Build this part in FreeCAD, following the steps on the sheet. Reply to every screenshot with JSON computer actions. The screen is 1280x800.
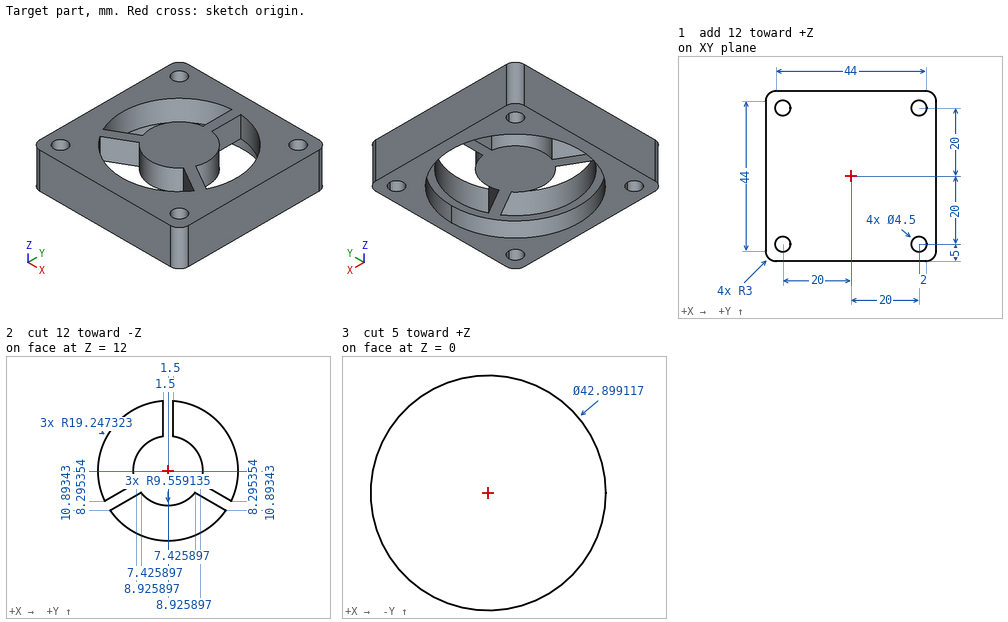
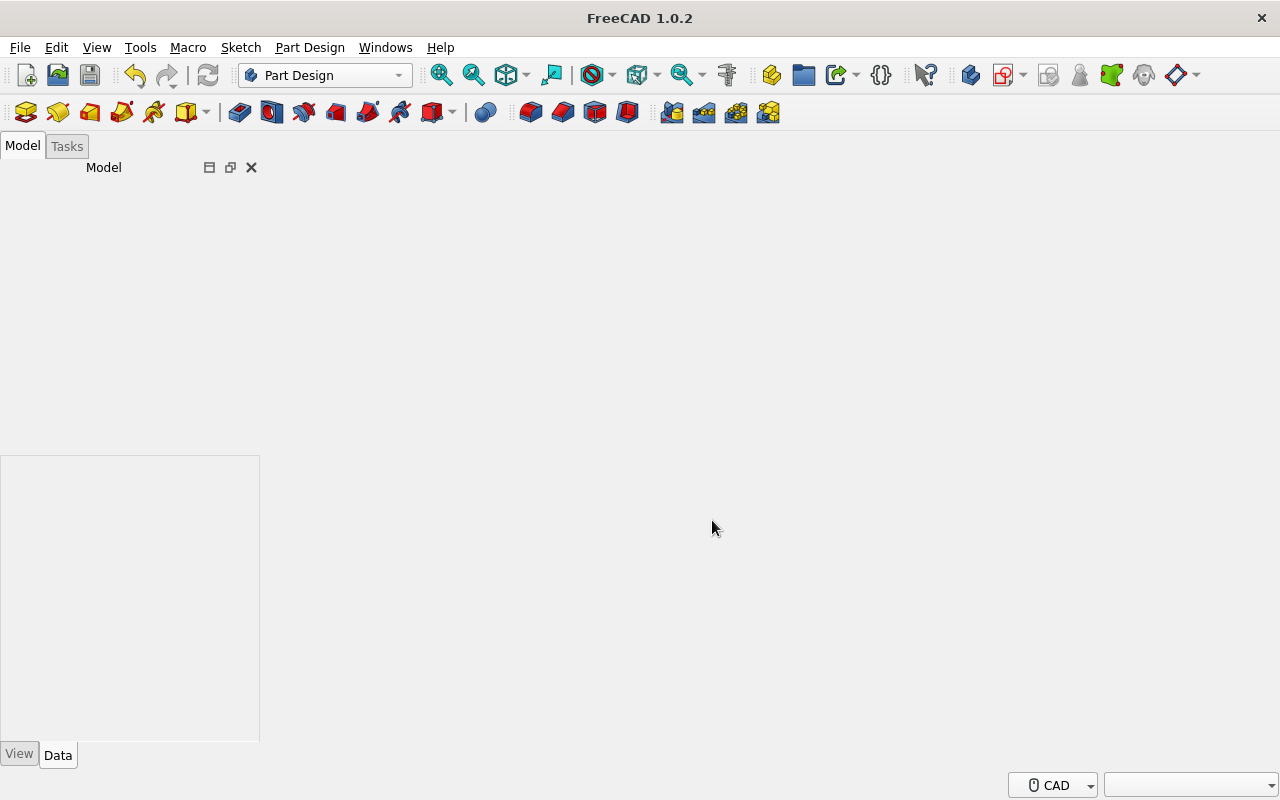
{"action": "left_click", "coordinate": [26, 76]}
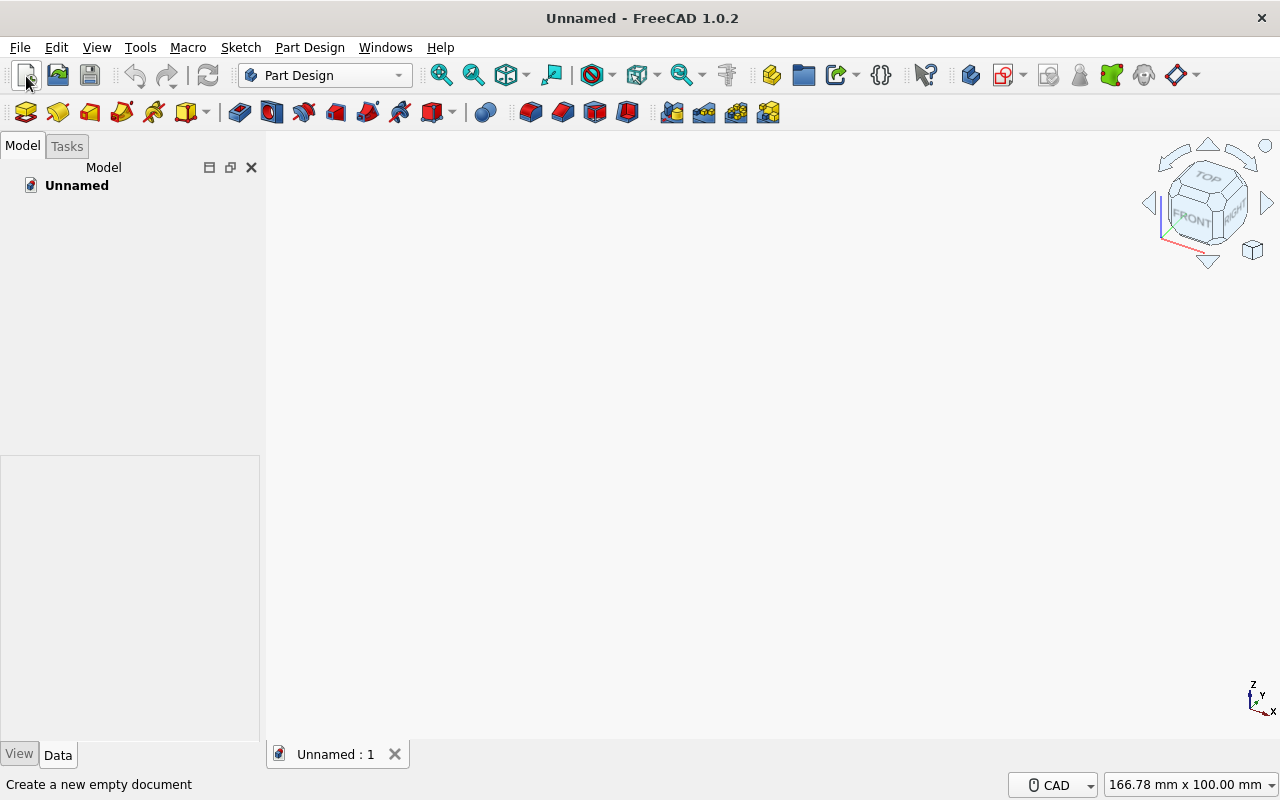
{"action": "left_click", "coordinate": [1004, 76]}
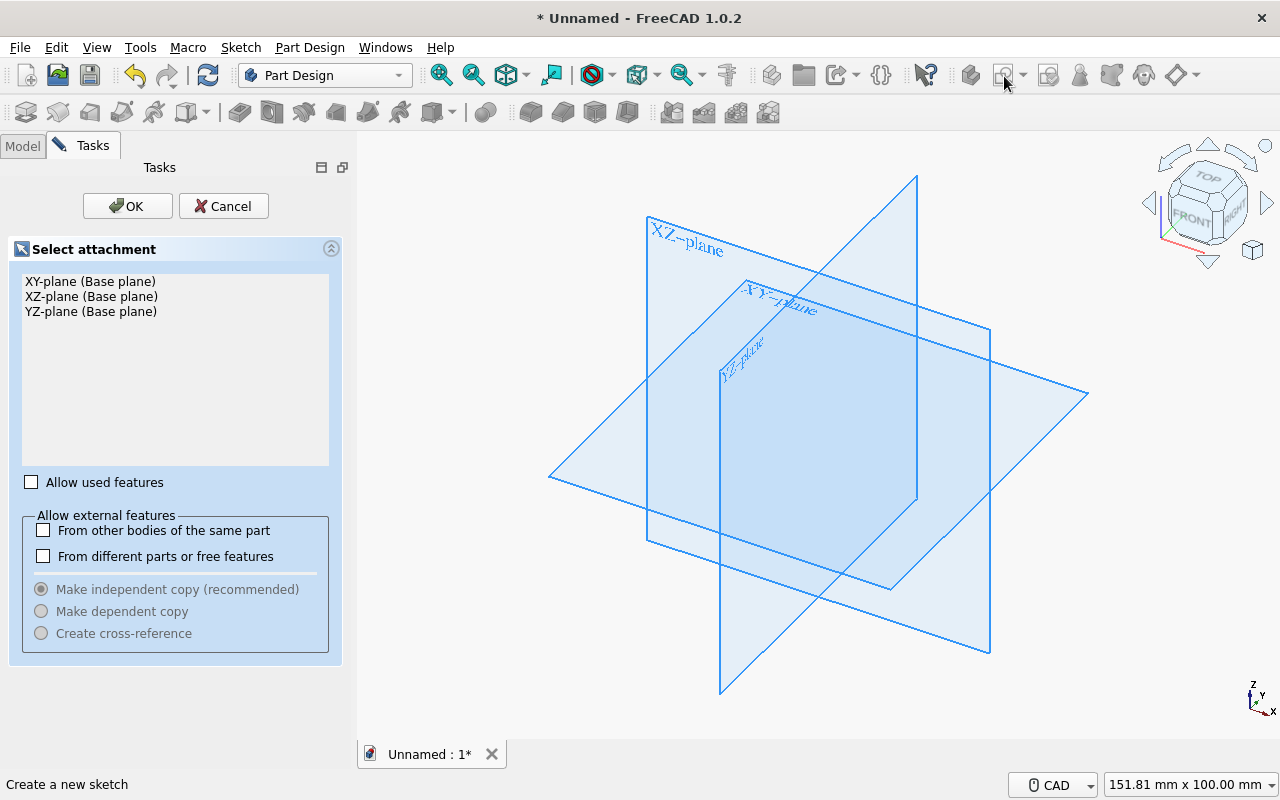
{"action": "left_click", "coordinate": [82, 282]}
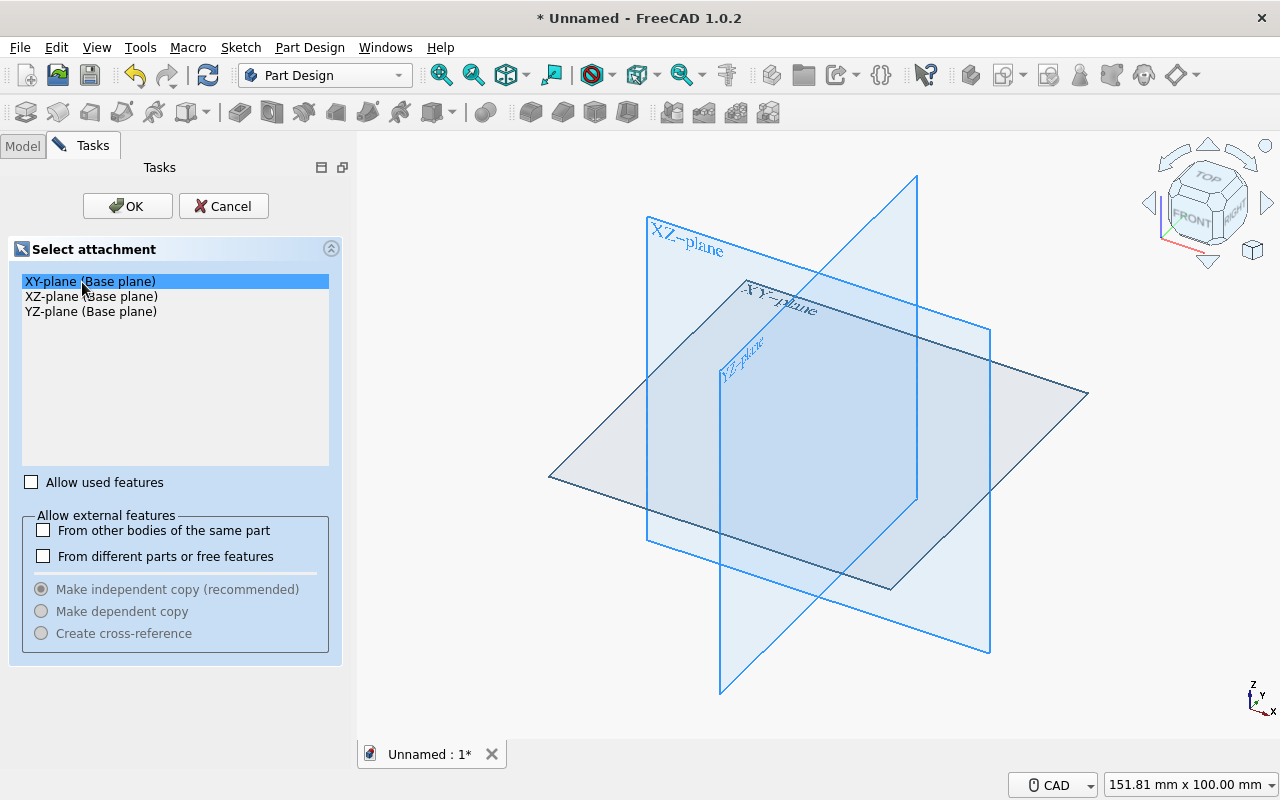
{"action": "left_click", "coordinate": [128, 206]}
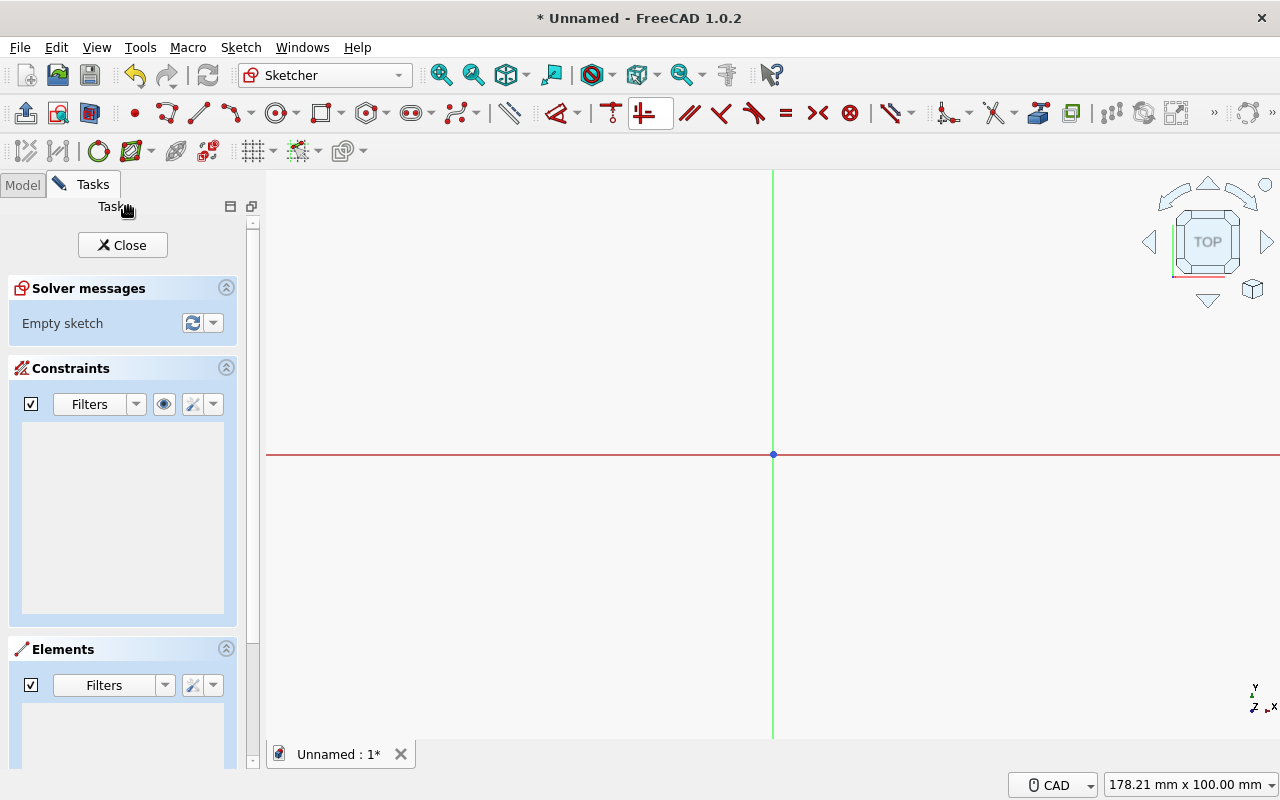
{"action": "left_click", "coordinate": [200, 114]}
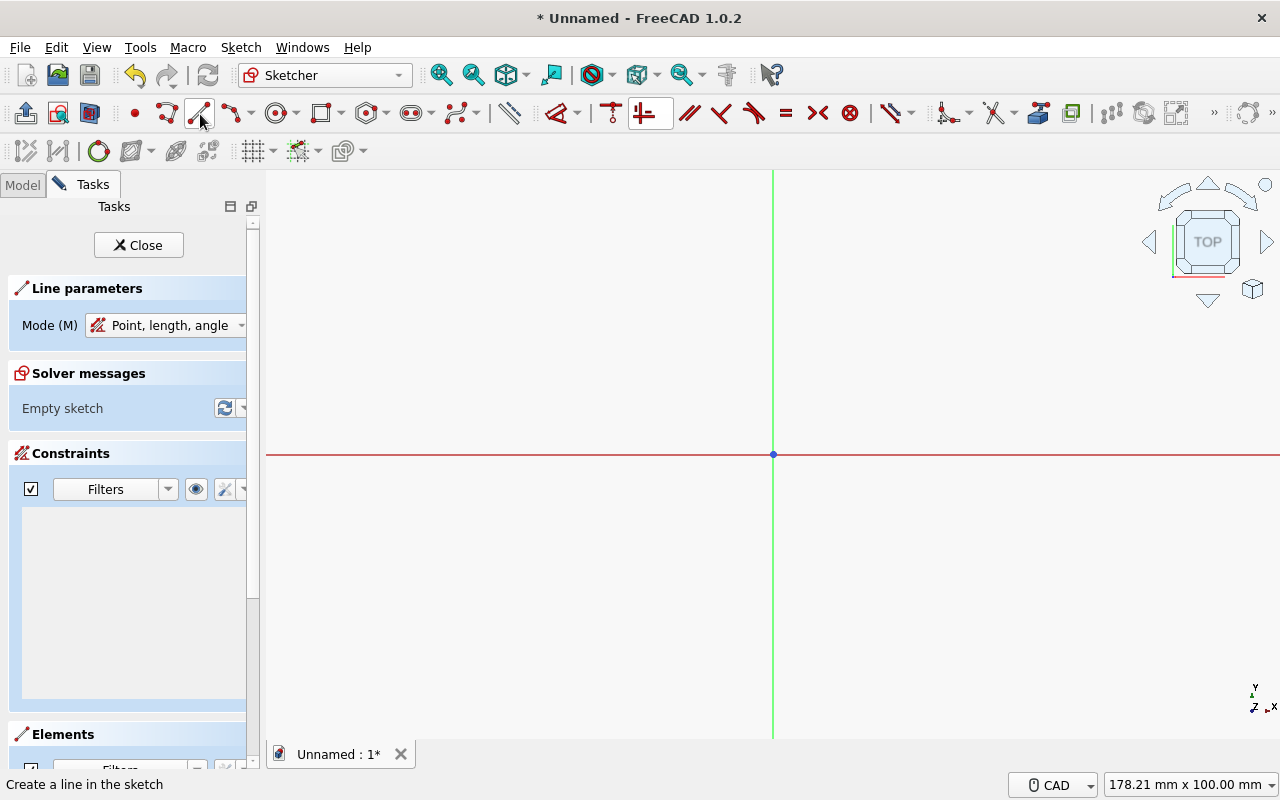
{"action": "left_click", "coordinate": [898, 312]}
{"action": "left_click", "coordinate": [648, 312]}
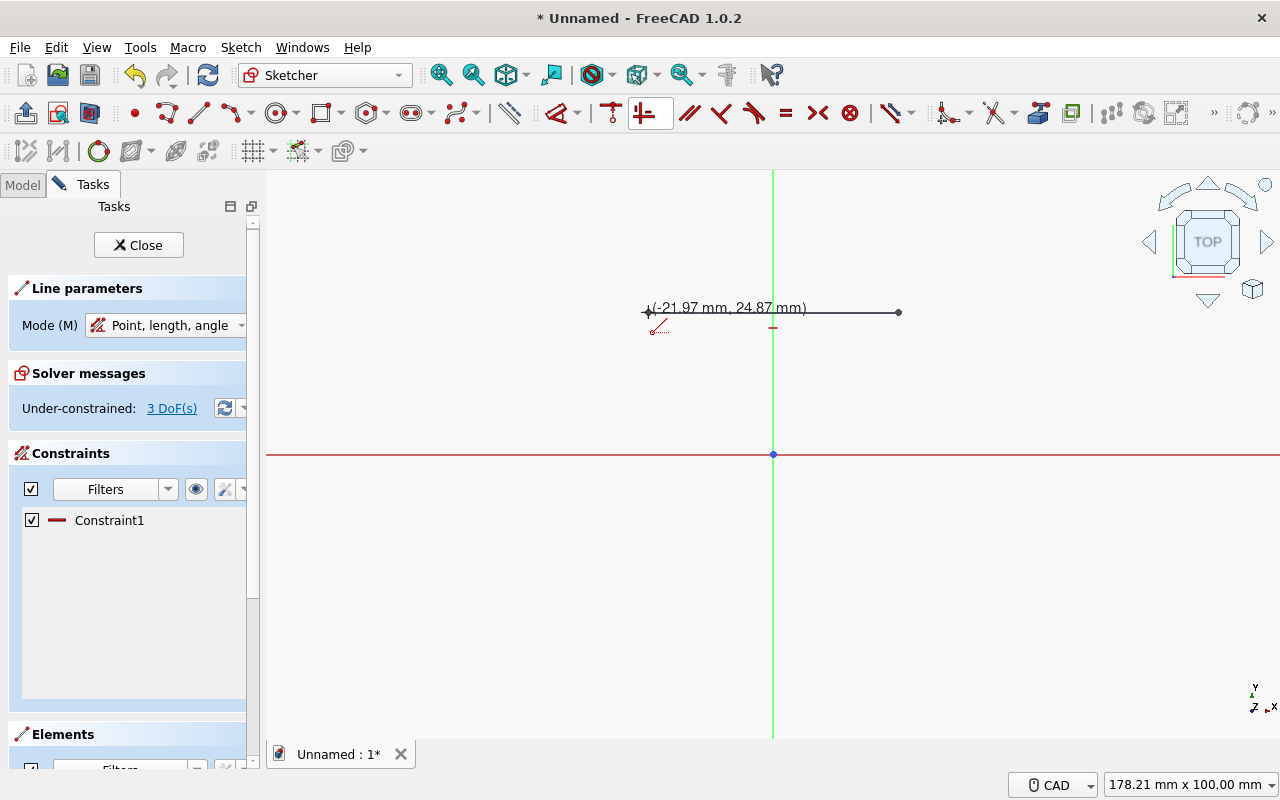
{"action": "left_click", "coordinate": [631, 329]}
{"action": "left_click", "coordinate": [631, 580]}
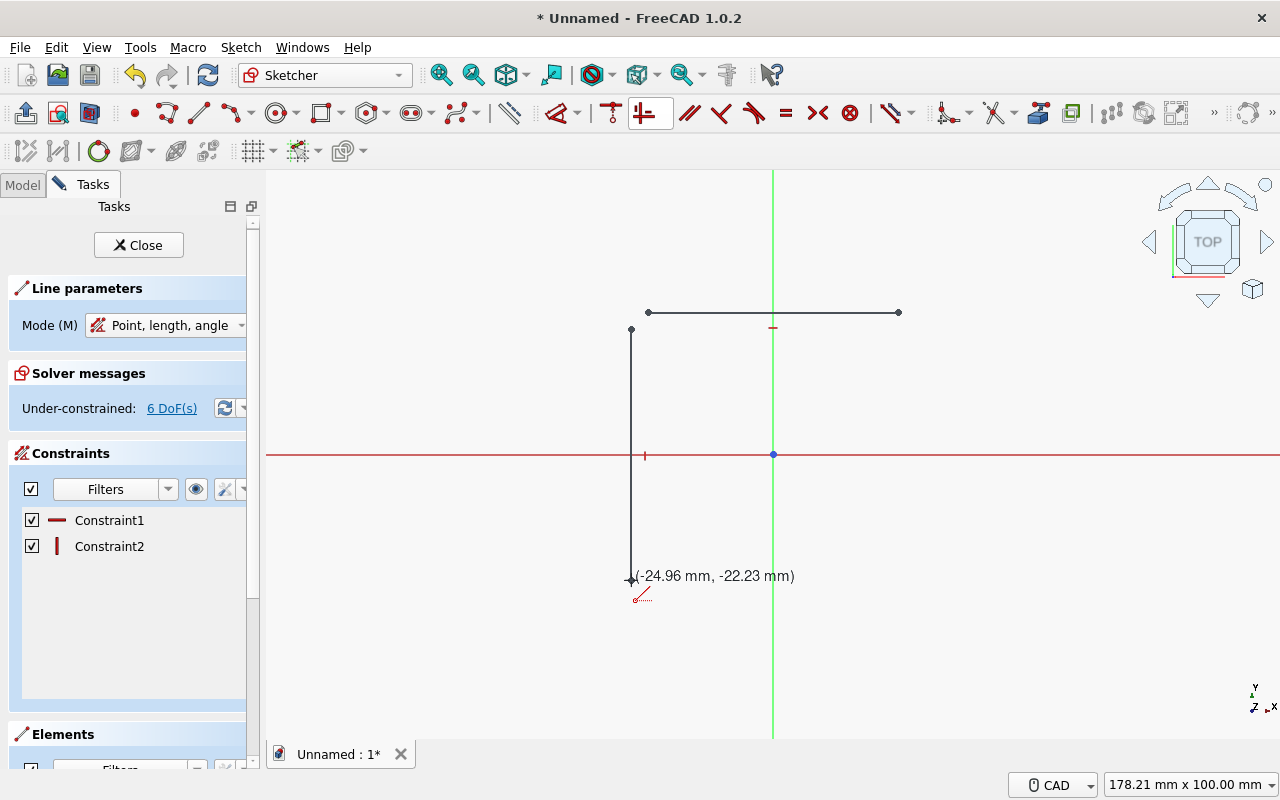
{"action": "left_click", "coordinate": [648, 597]}
{"action": "left_click", "coordinate": [898, 597]}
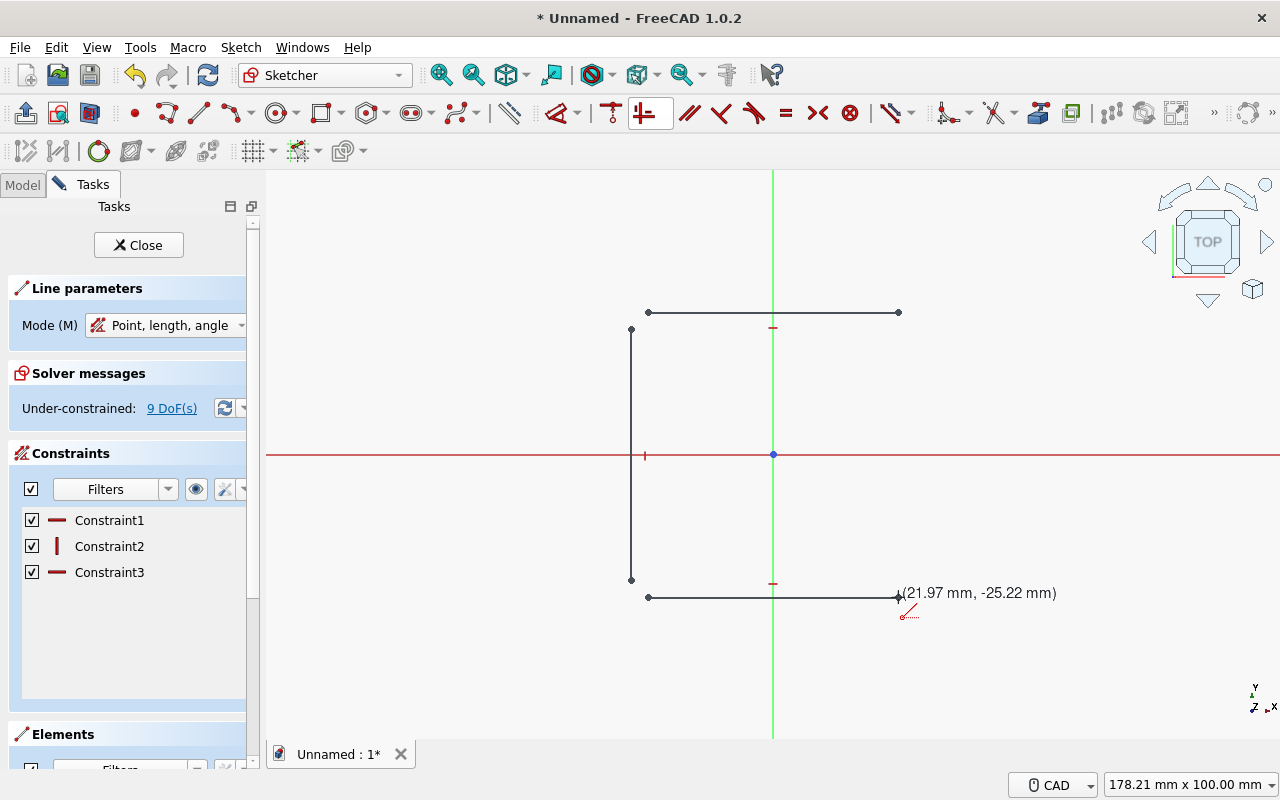
{"action": "left_click", "coordinate": [915, 580]}
{"action": "left_click", "coordinate": [915, 329]}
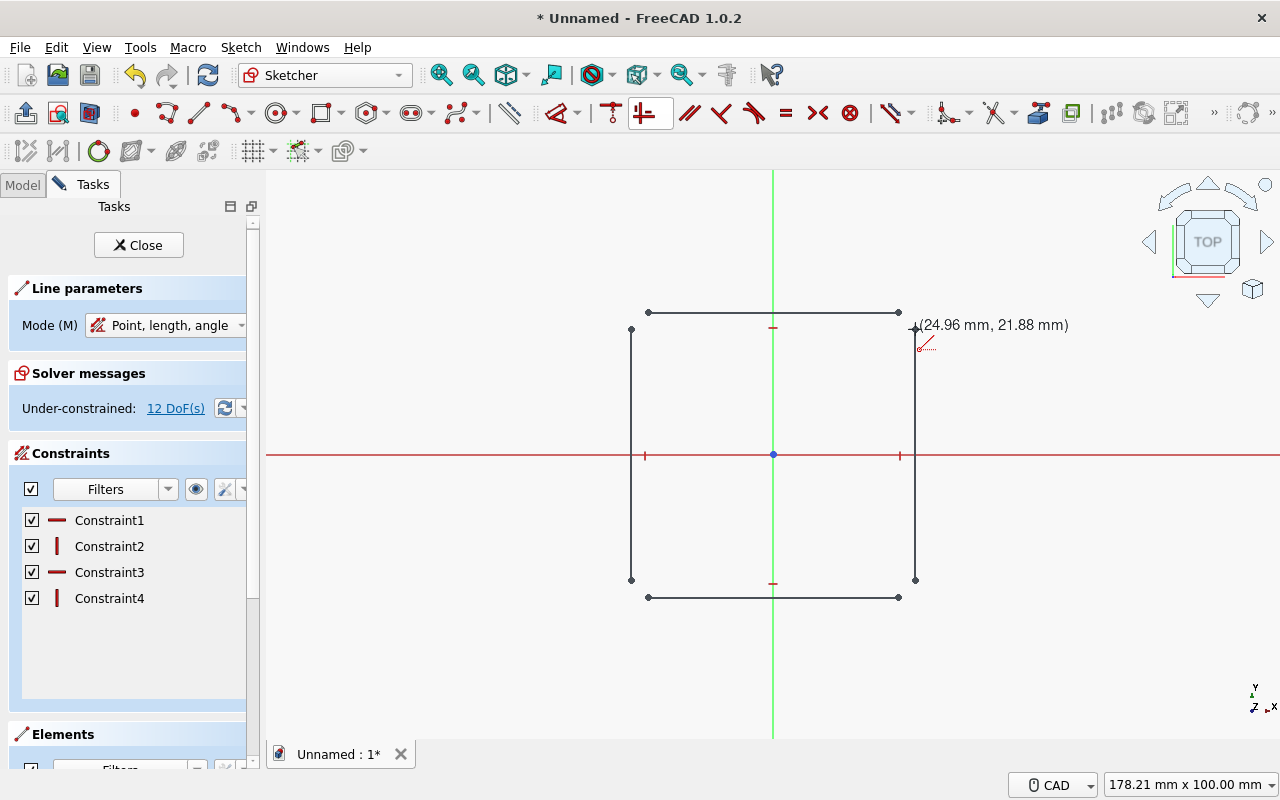
{"action": "left_click", "coordinate": [232, 114]}